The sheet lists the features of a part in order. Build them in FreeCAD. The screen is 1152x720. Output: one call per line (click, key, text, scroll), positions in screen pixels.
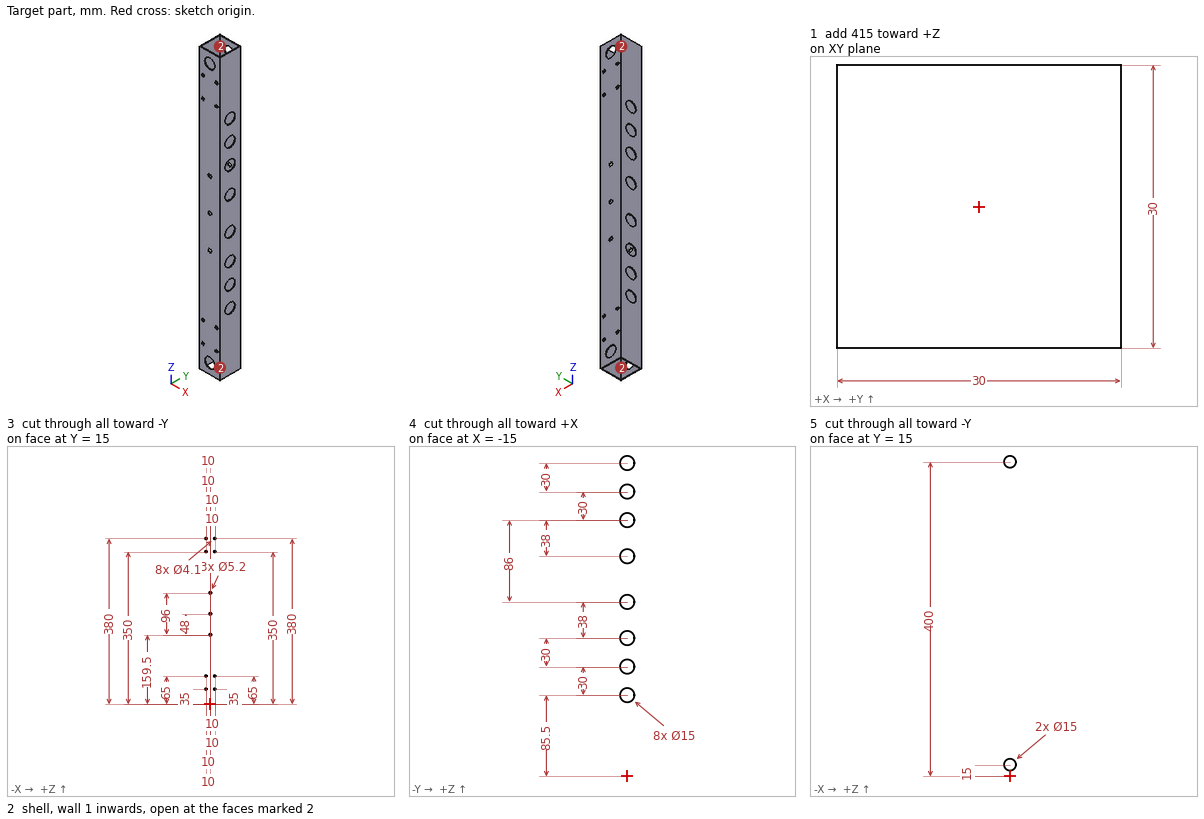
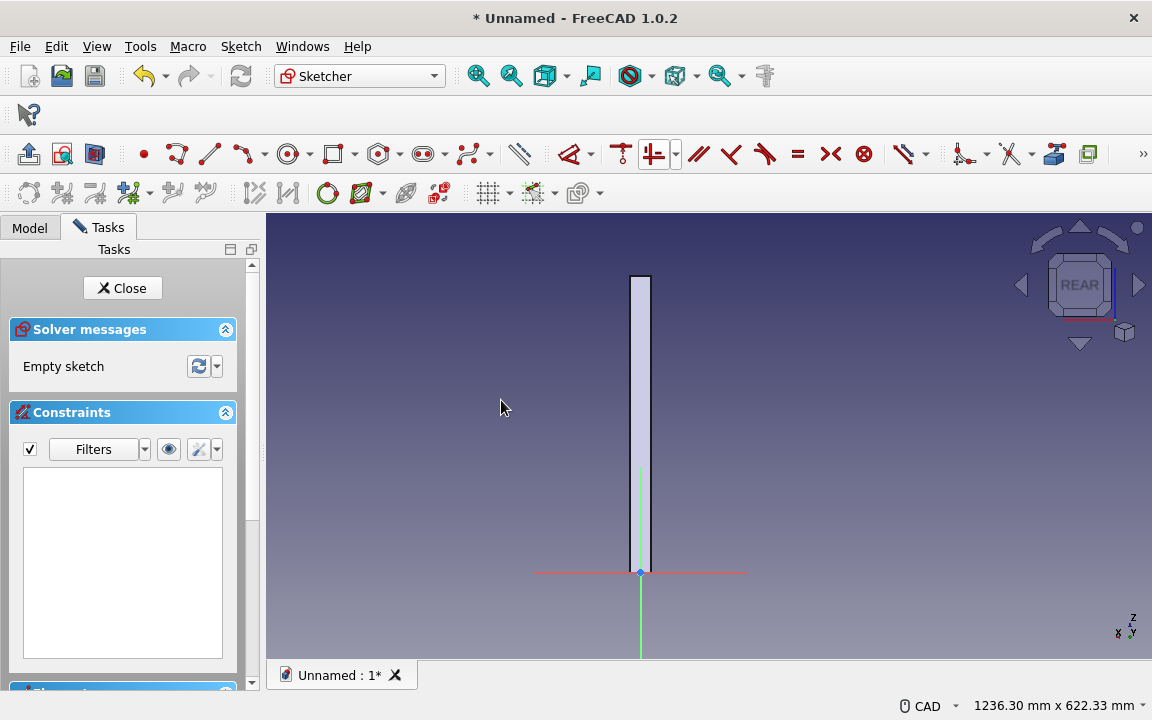
click(288, 154)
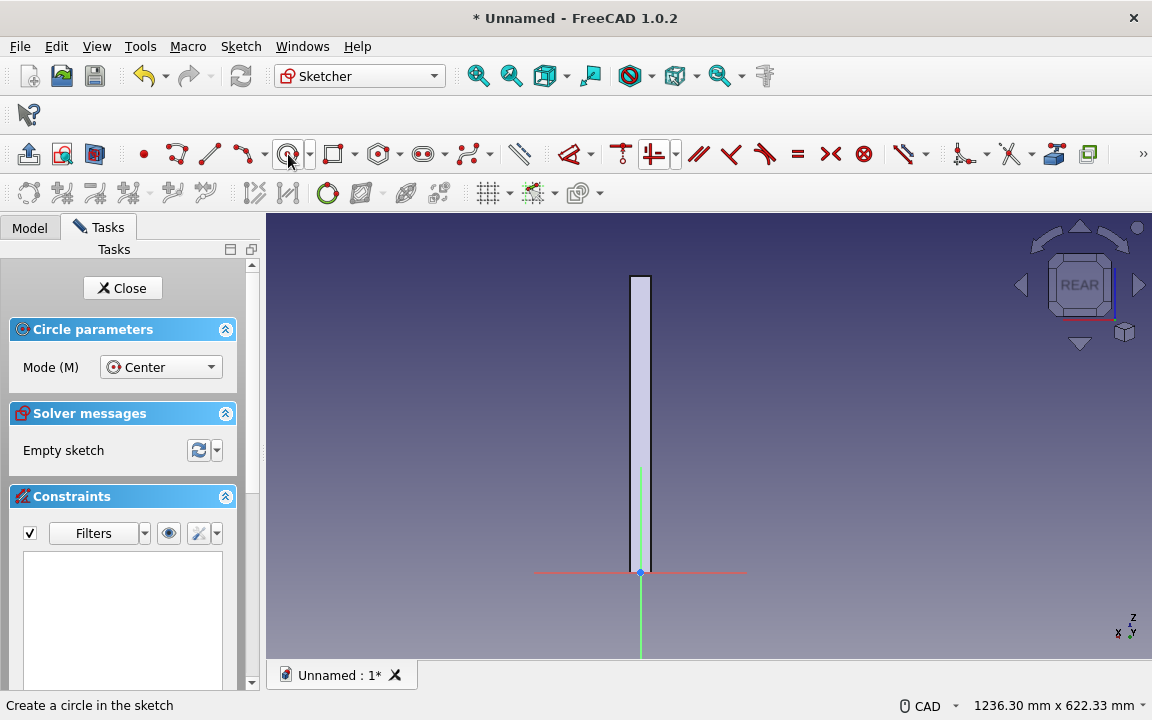
scroll(641, 459, up, 13)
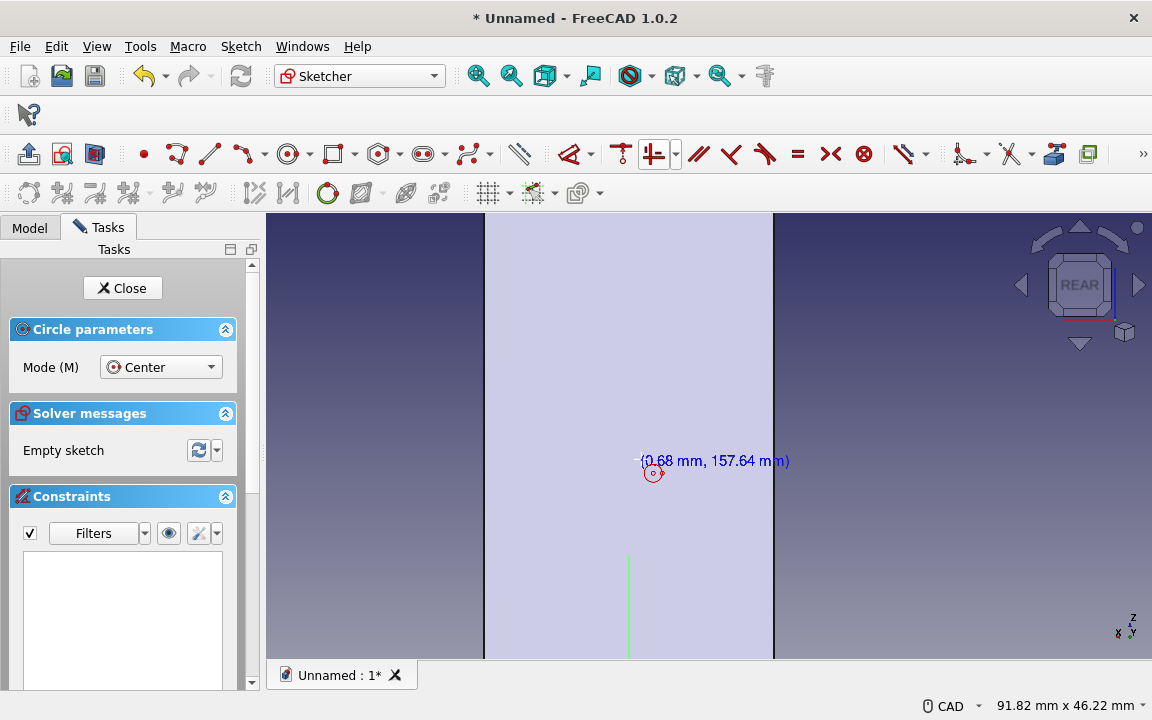
scroll(641, 459, down, 13)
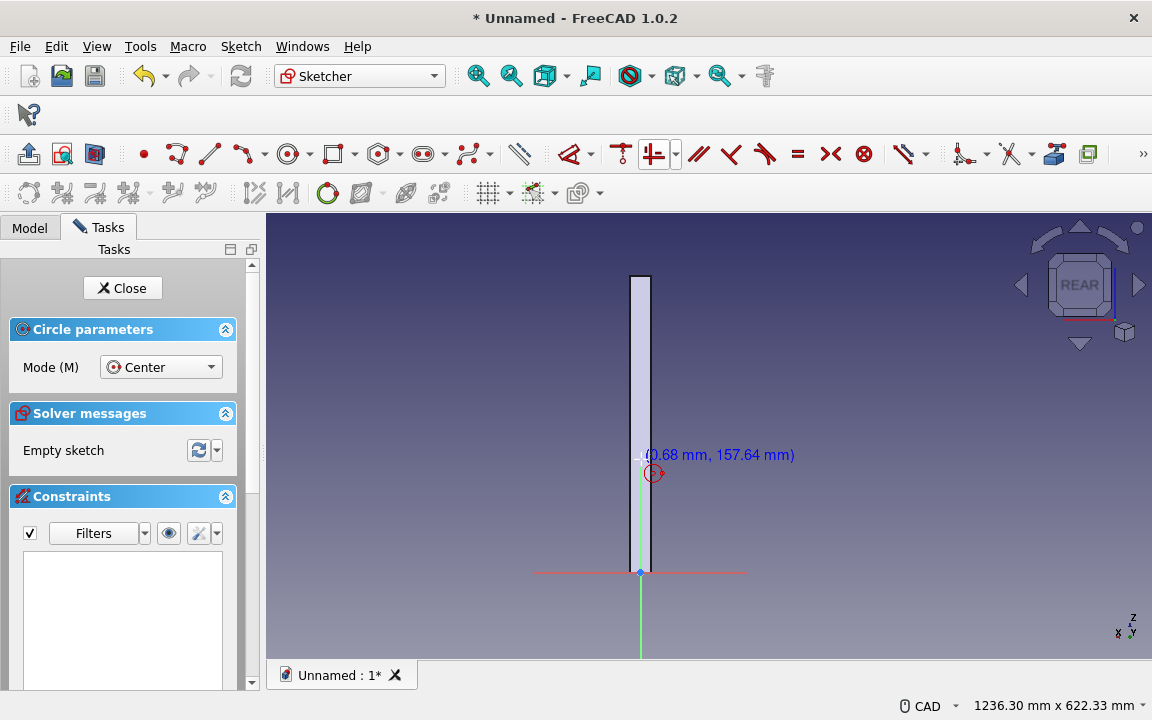
click(641, 459)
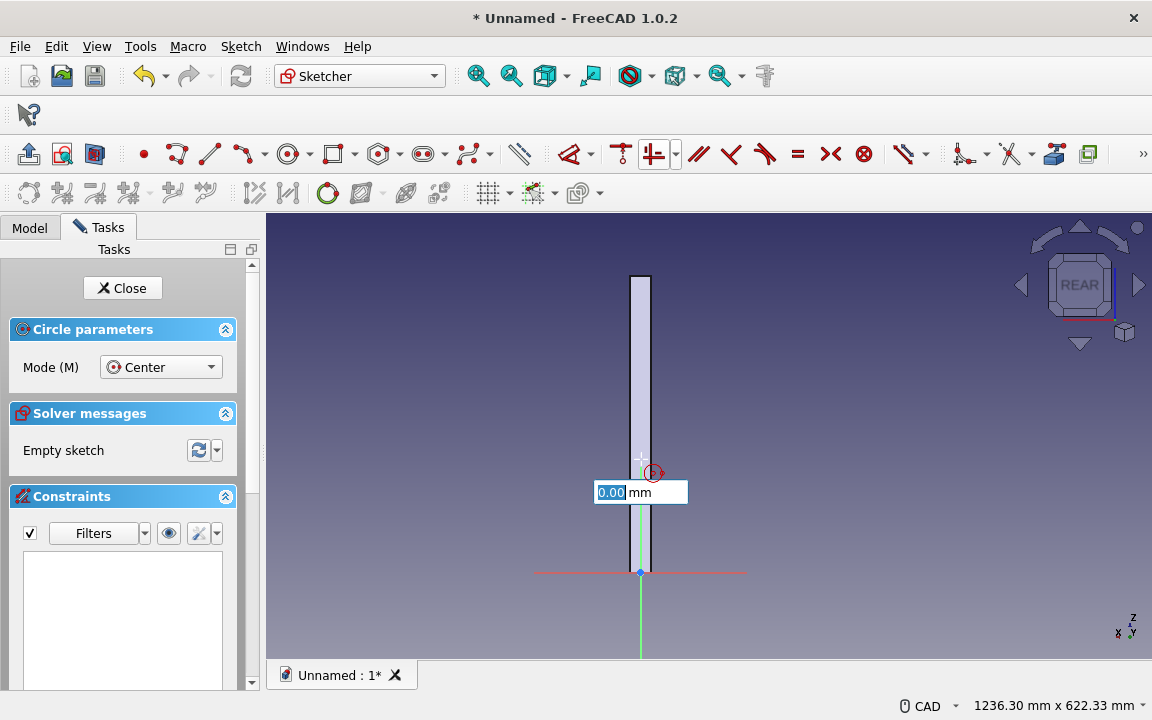
scroll(642, 458, up, 12)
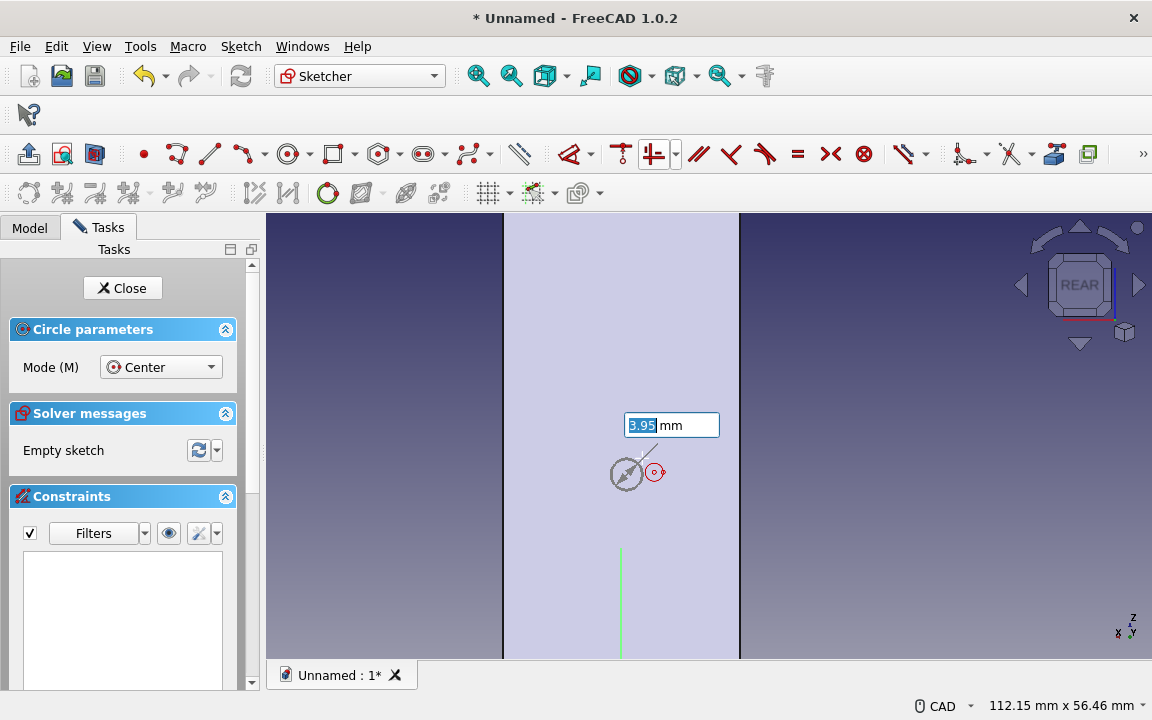
click(641, 453)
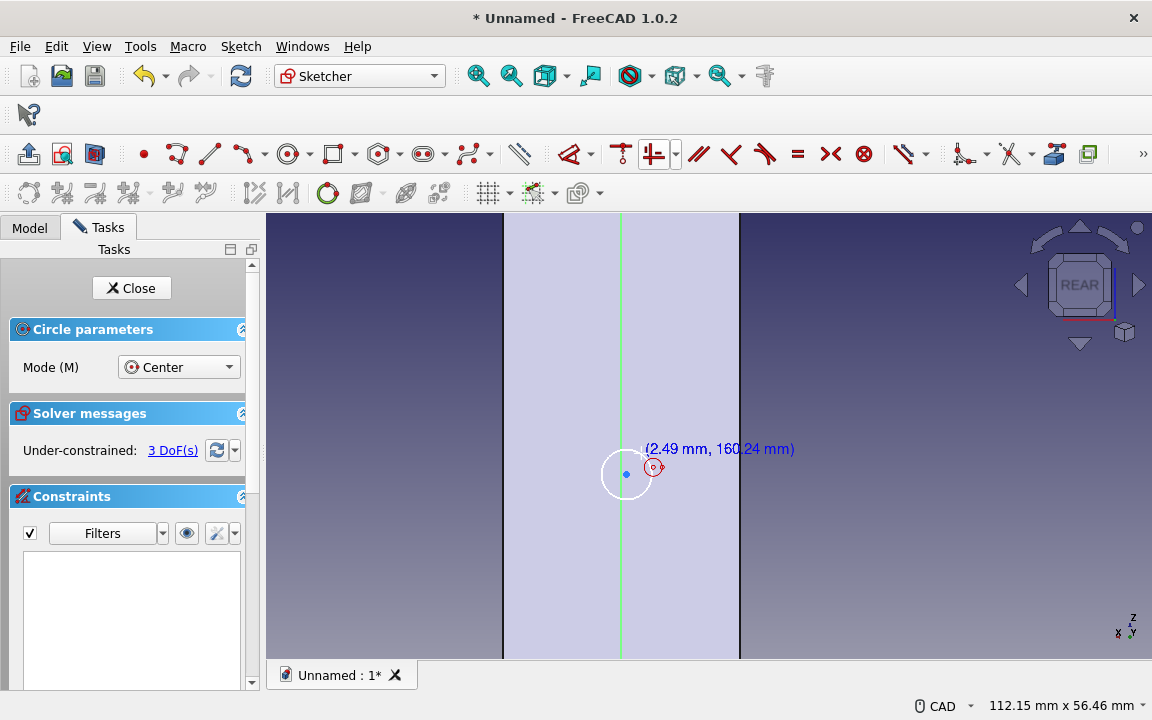
scroll(642, 458, down, 12)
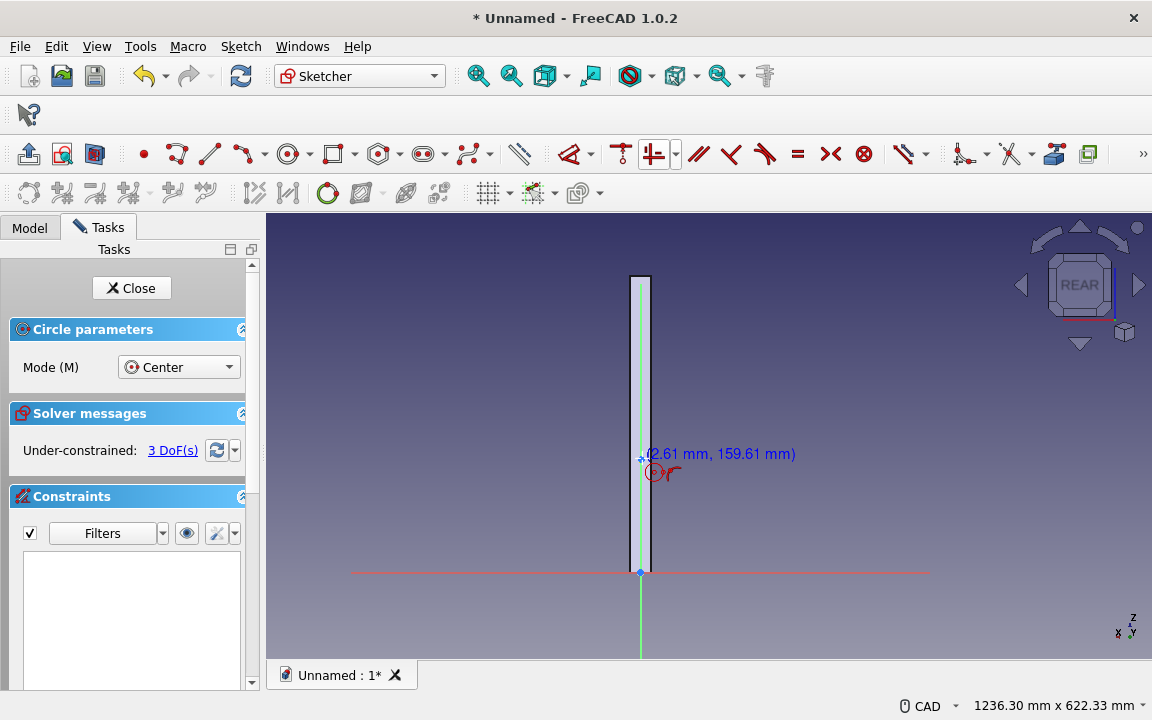
scroll(641, 390, up, 13)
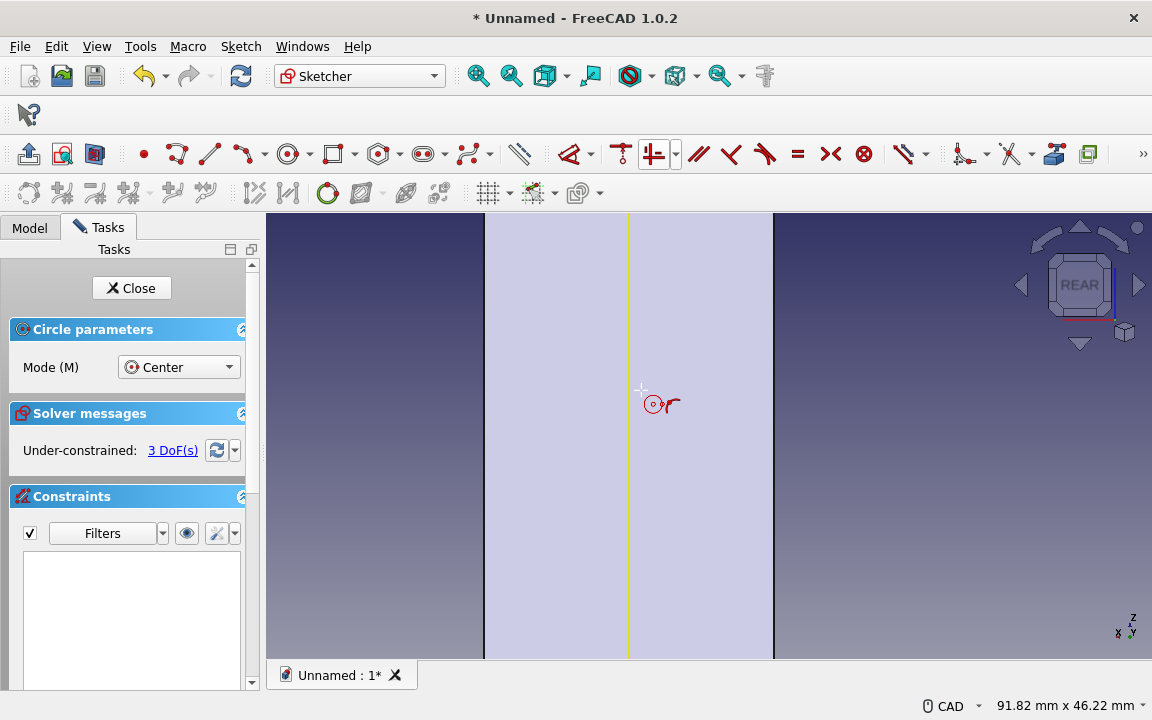
scroll(641, 390, down, 13)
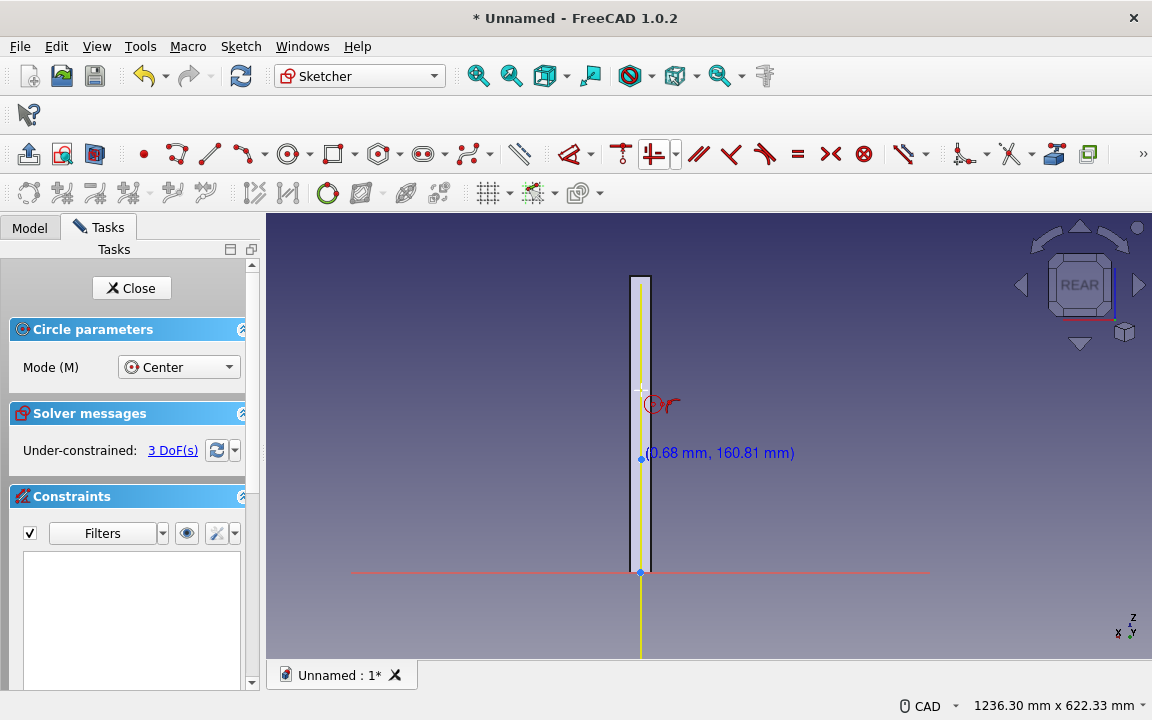
click(641, 390)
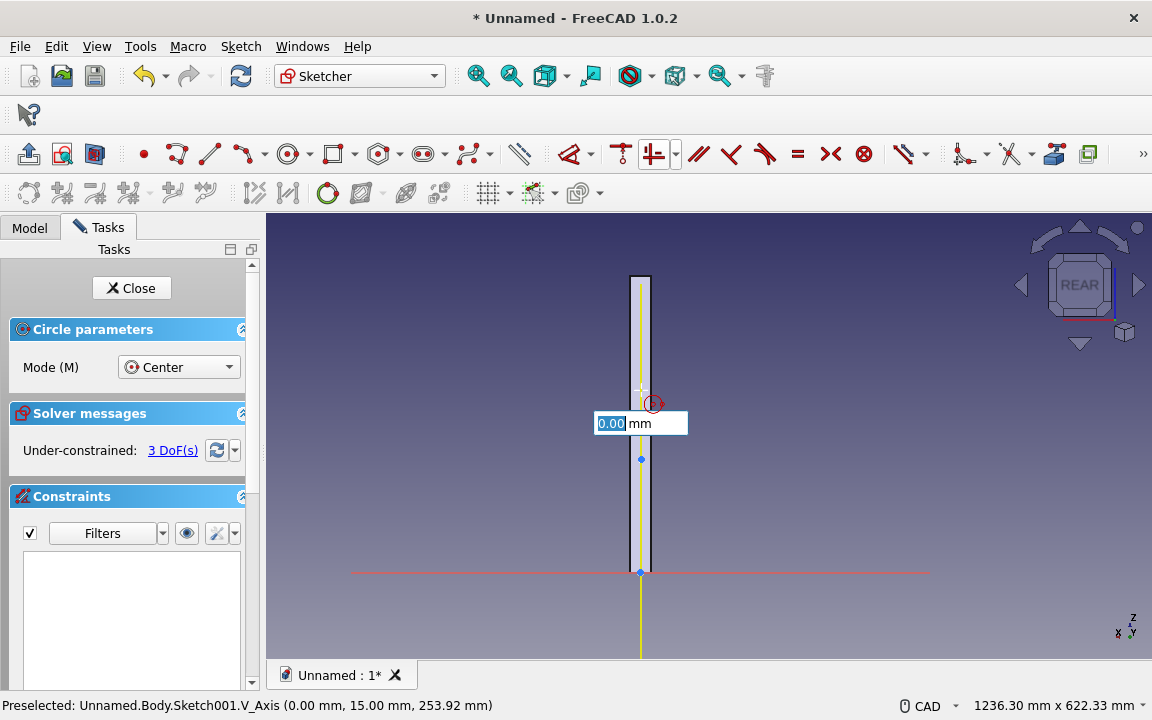
scroll(642, 389, up, 12)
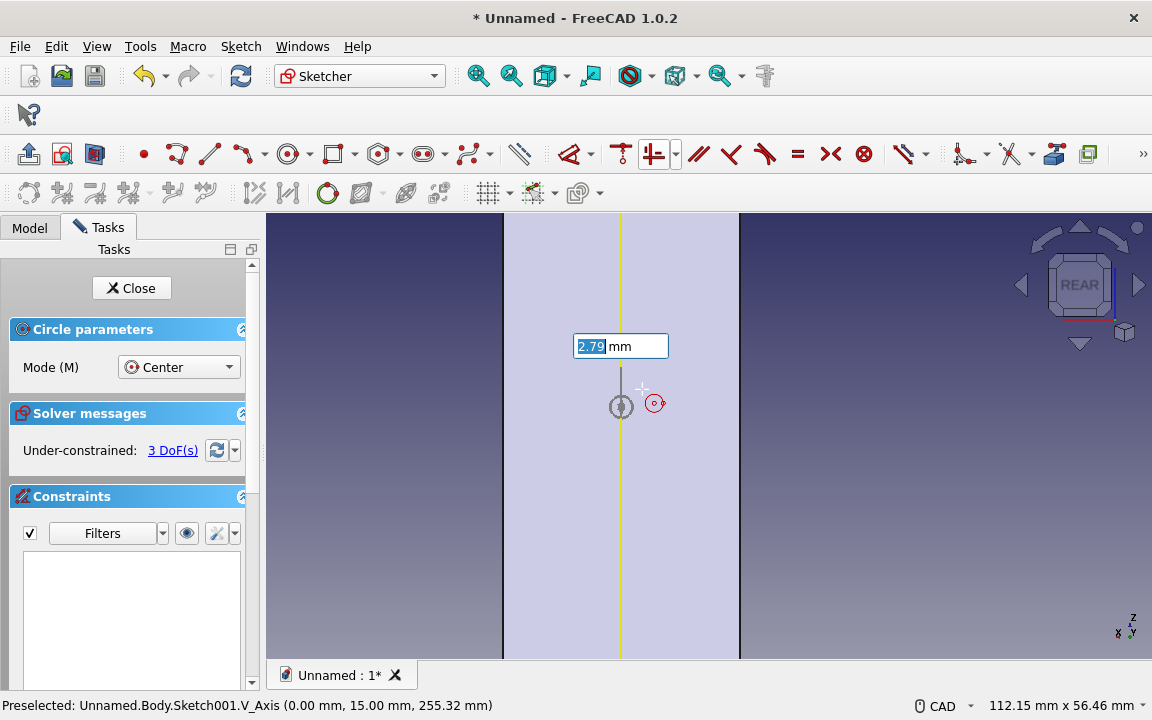
click(641, 388)